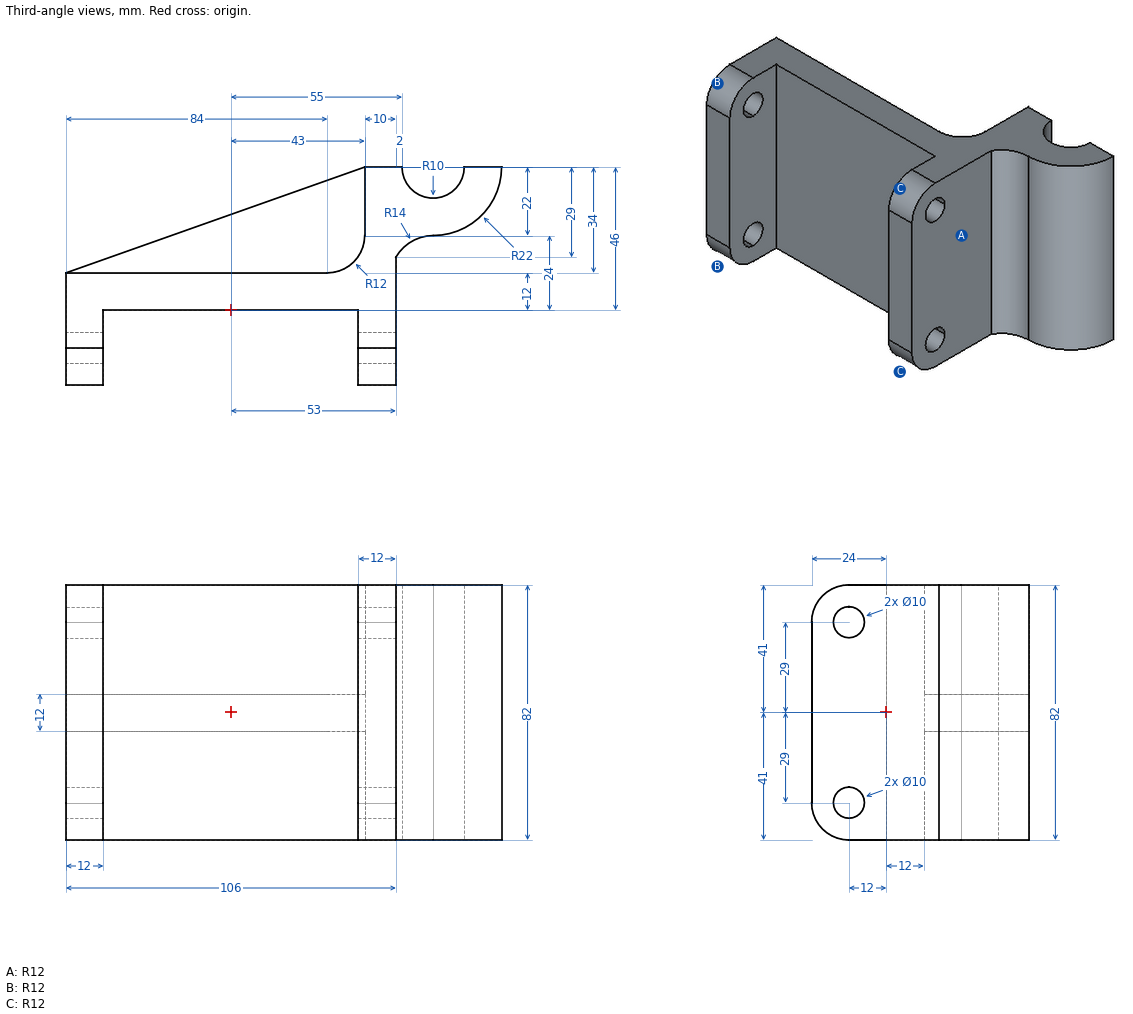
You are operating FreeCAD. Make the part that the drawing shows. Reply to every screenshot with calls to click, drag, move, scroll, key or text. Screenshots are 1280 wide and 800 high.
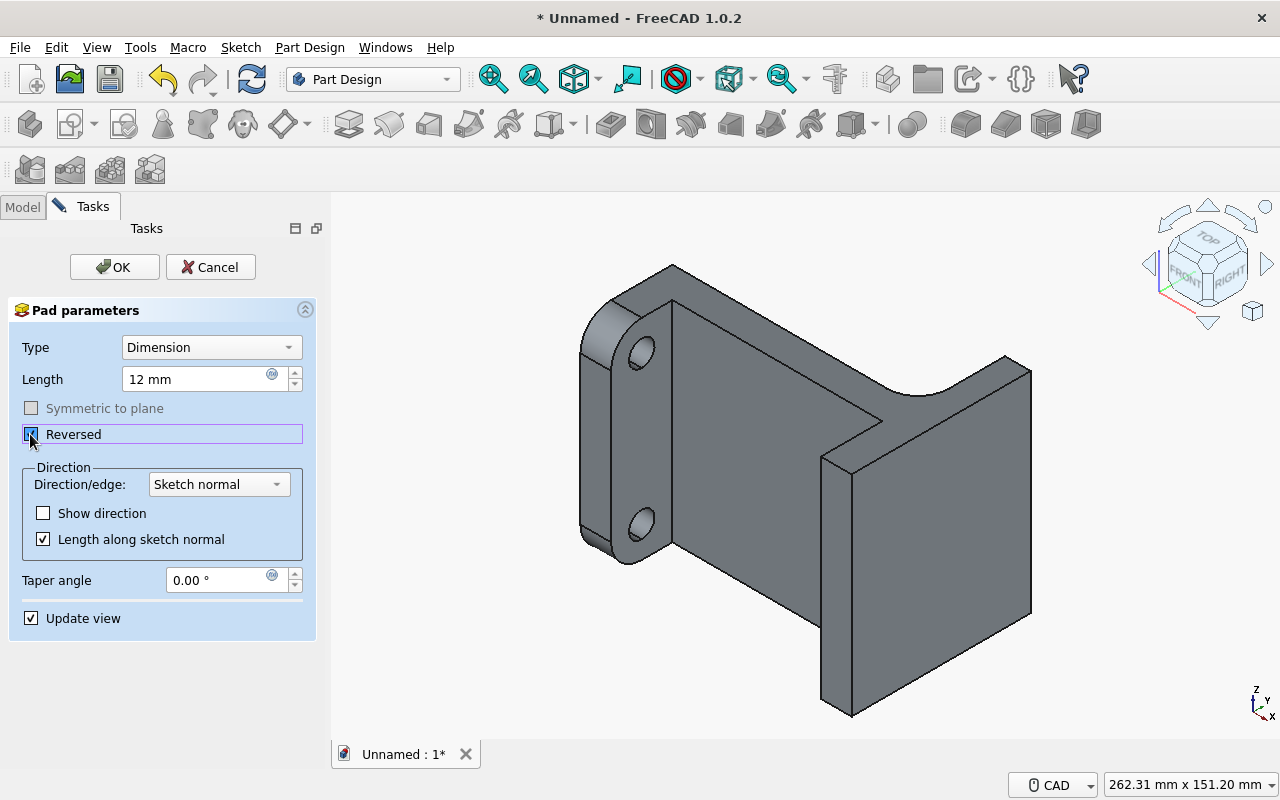
click(115, 267)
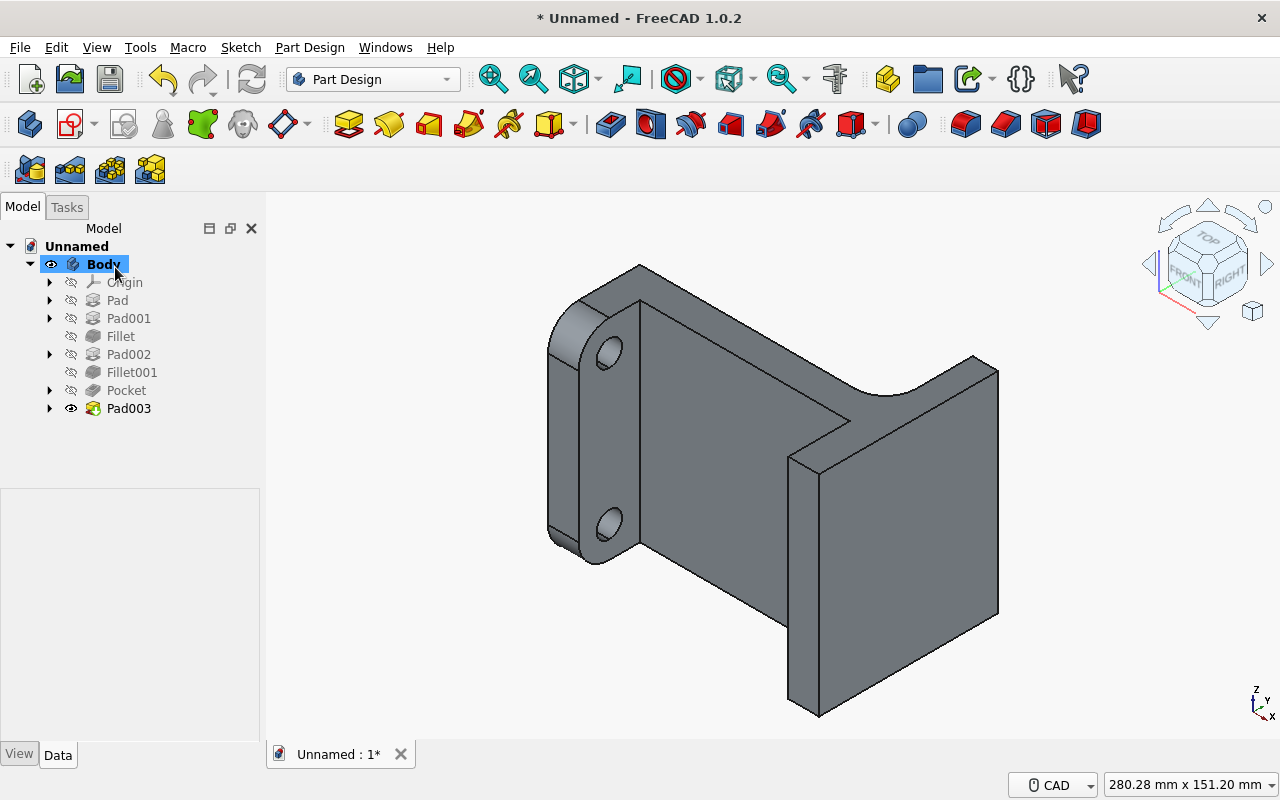
click(804, 464)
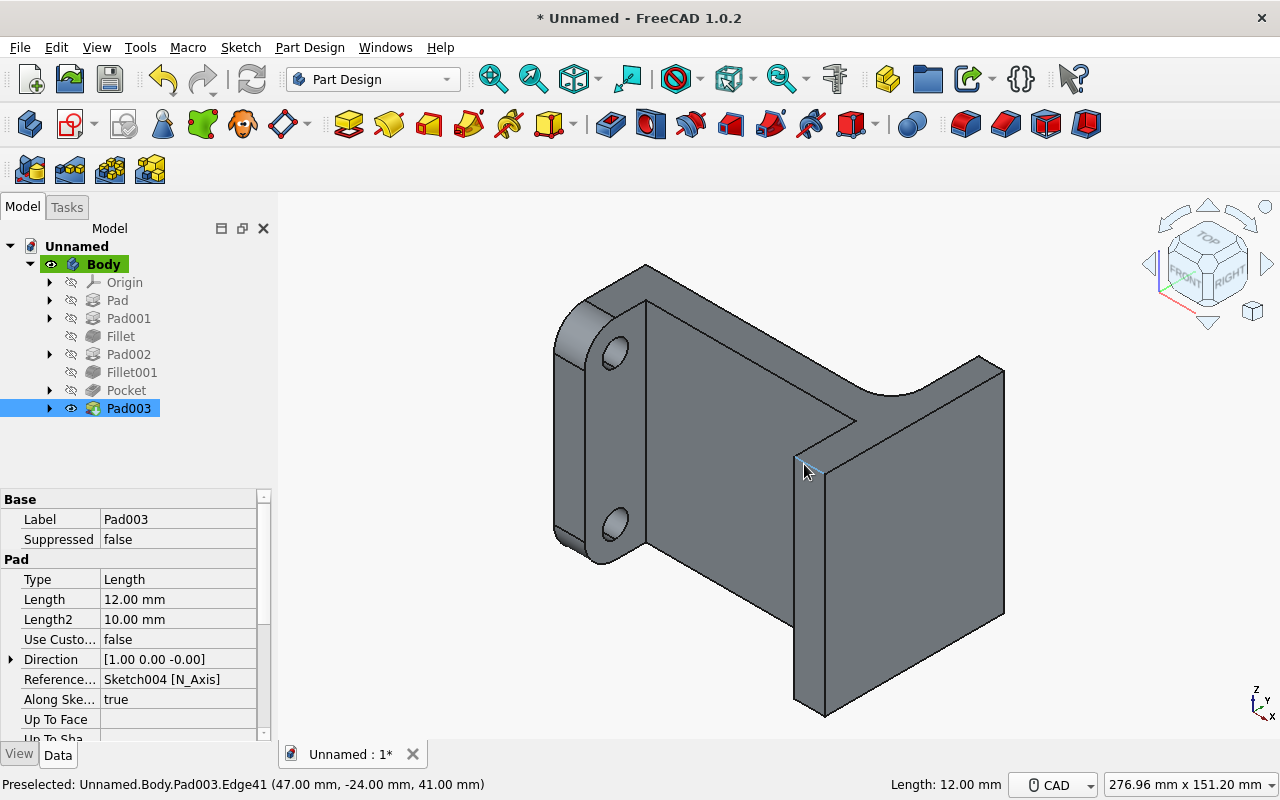
key(2)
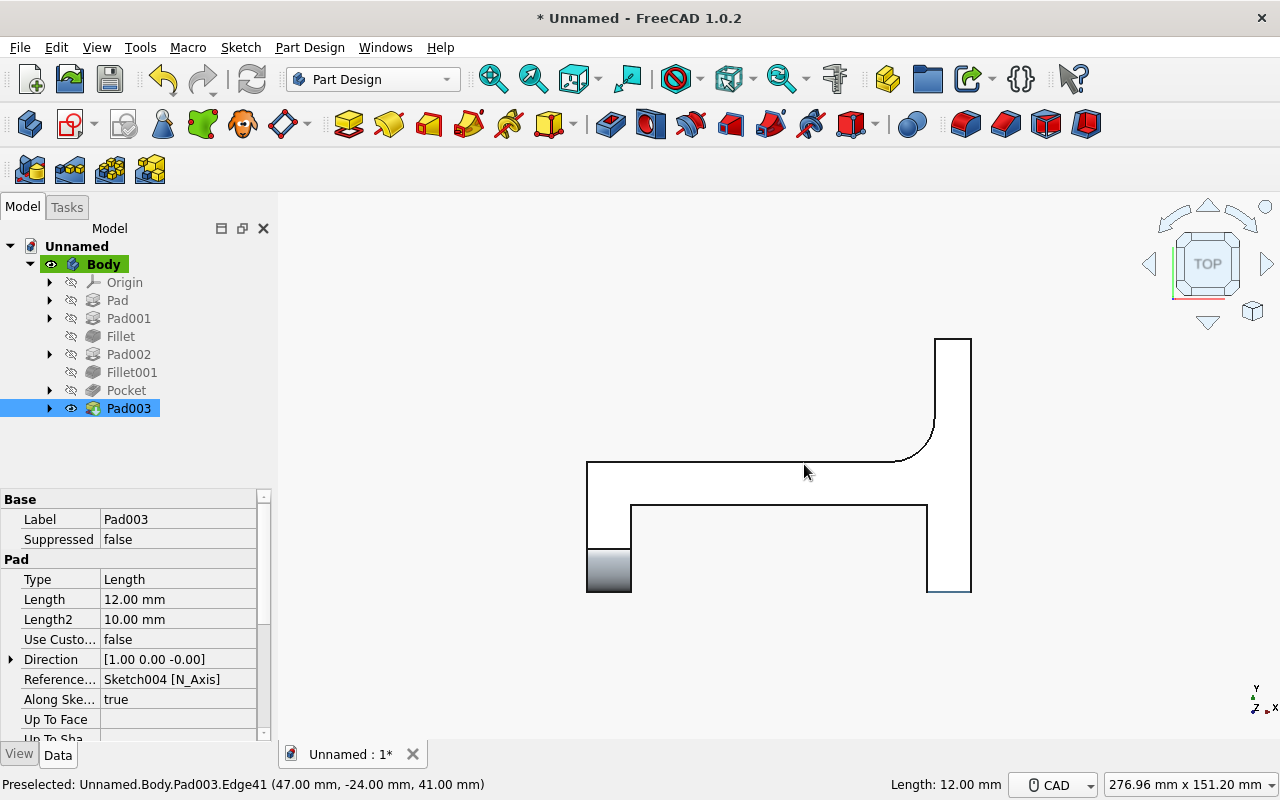
key(0)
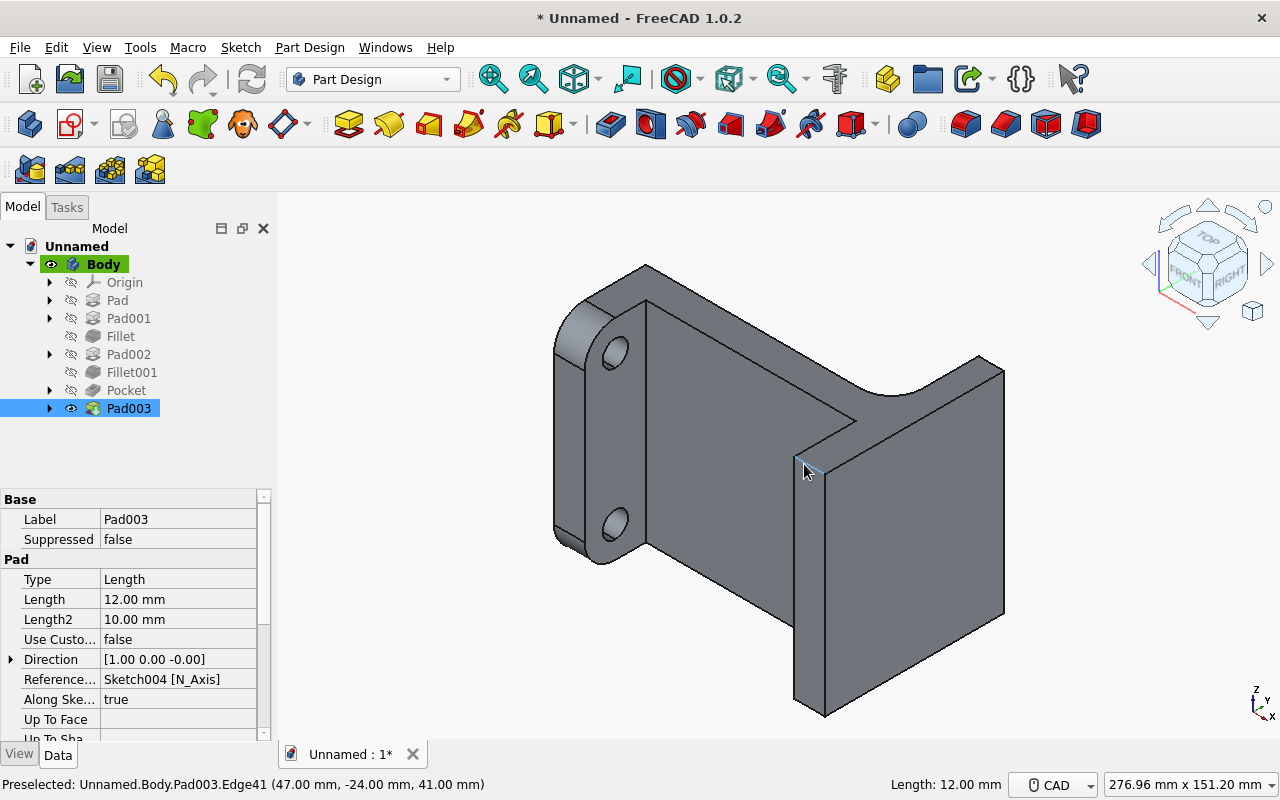
key(1)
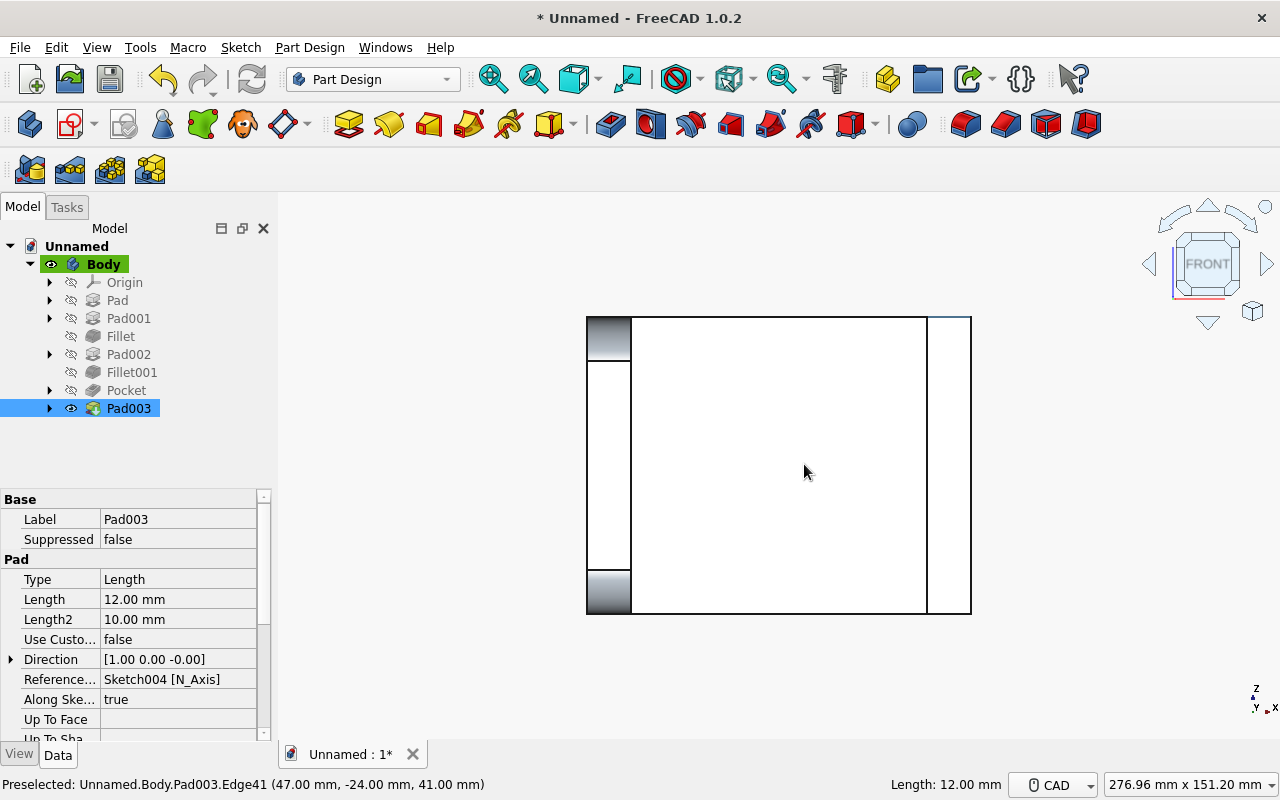
key(3)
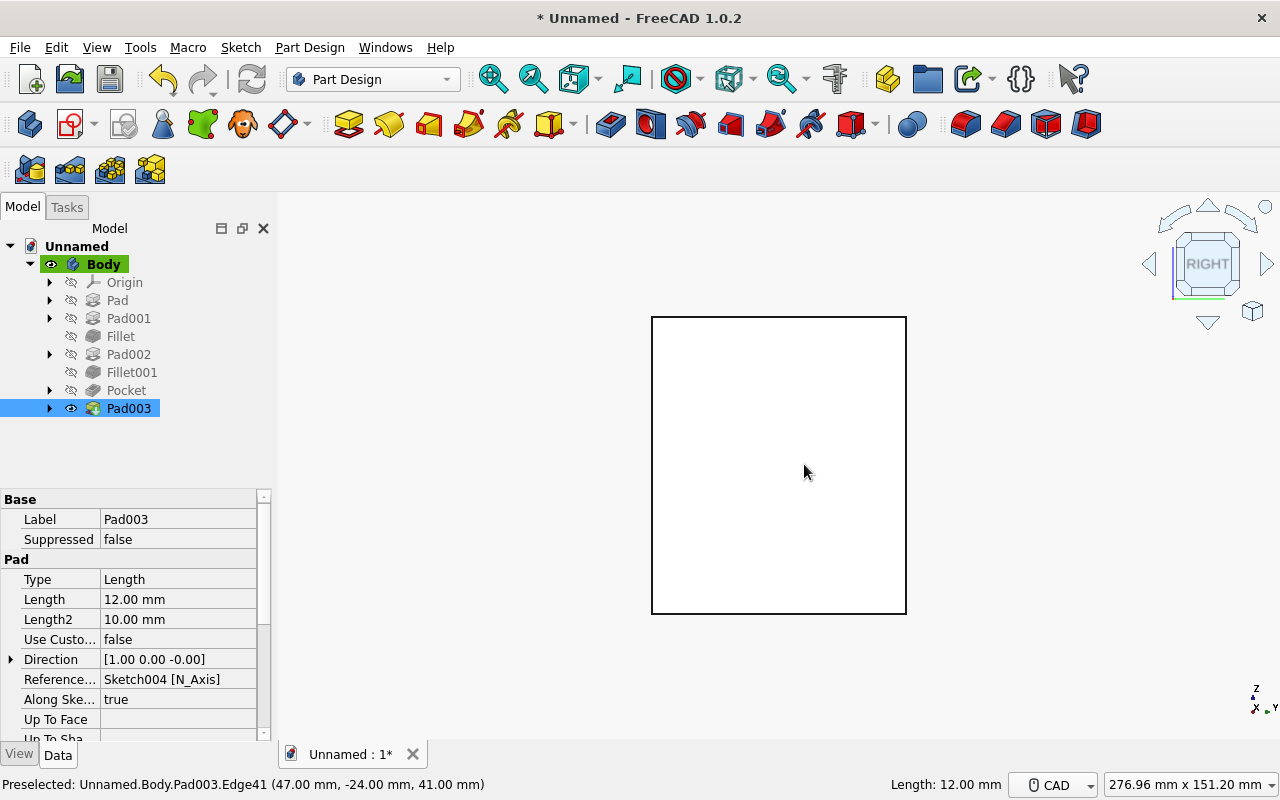
key(5)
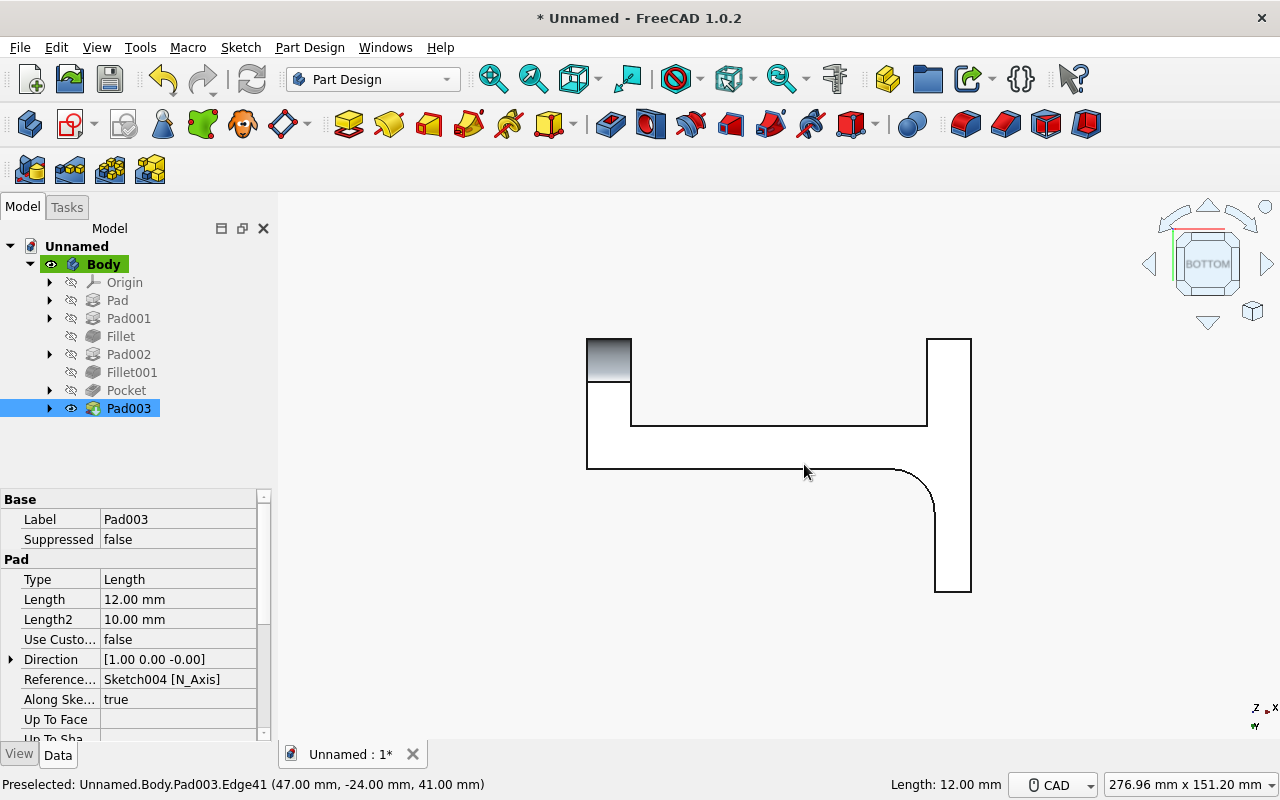
click(949, 338, ctrl)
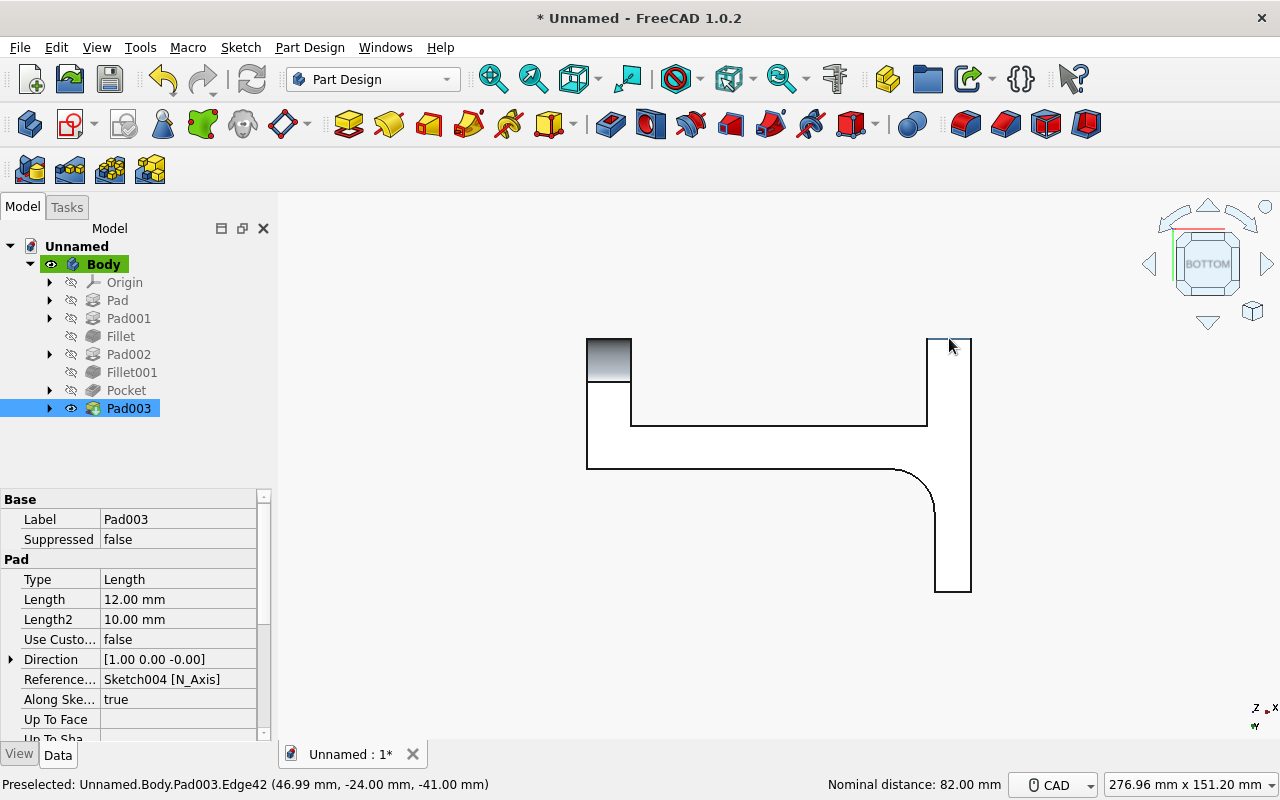
click(966, 124)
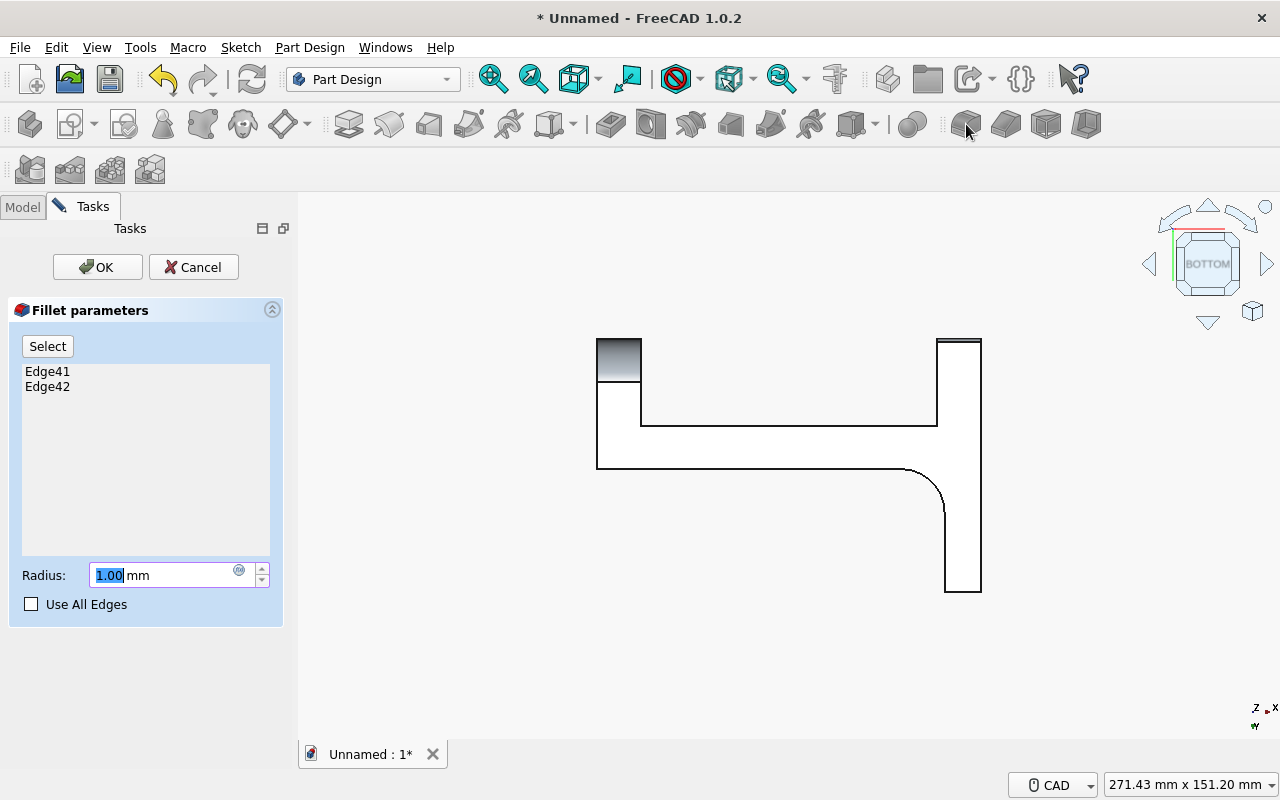
text(12)
key(Tab)